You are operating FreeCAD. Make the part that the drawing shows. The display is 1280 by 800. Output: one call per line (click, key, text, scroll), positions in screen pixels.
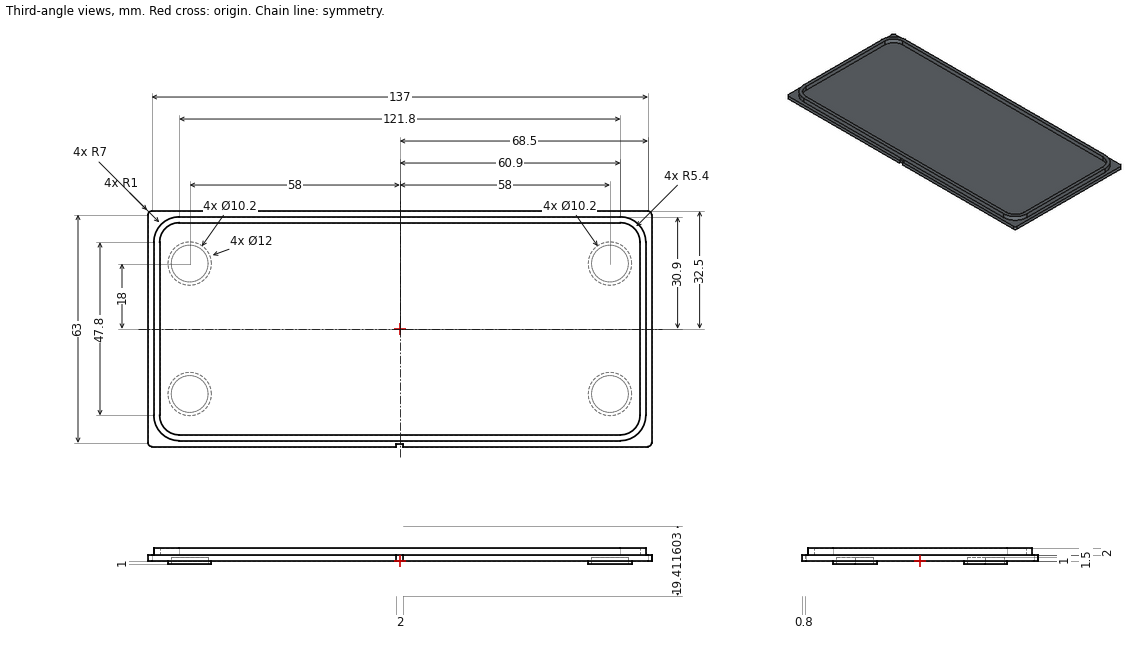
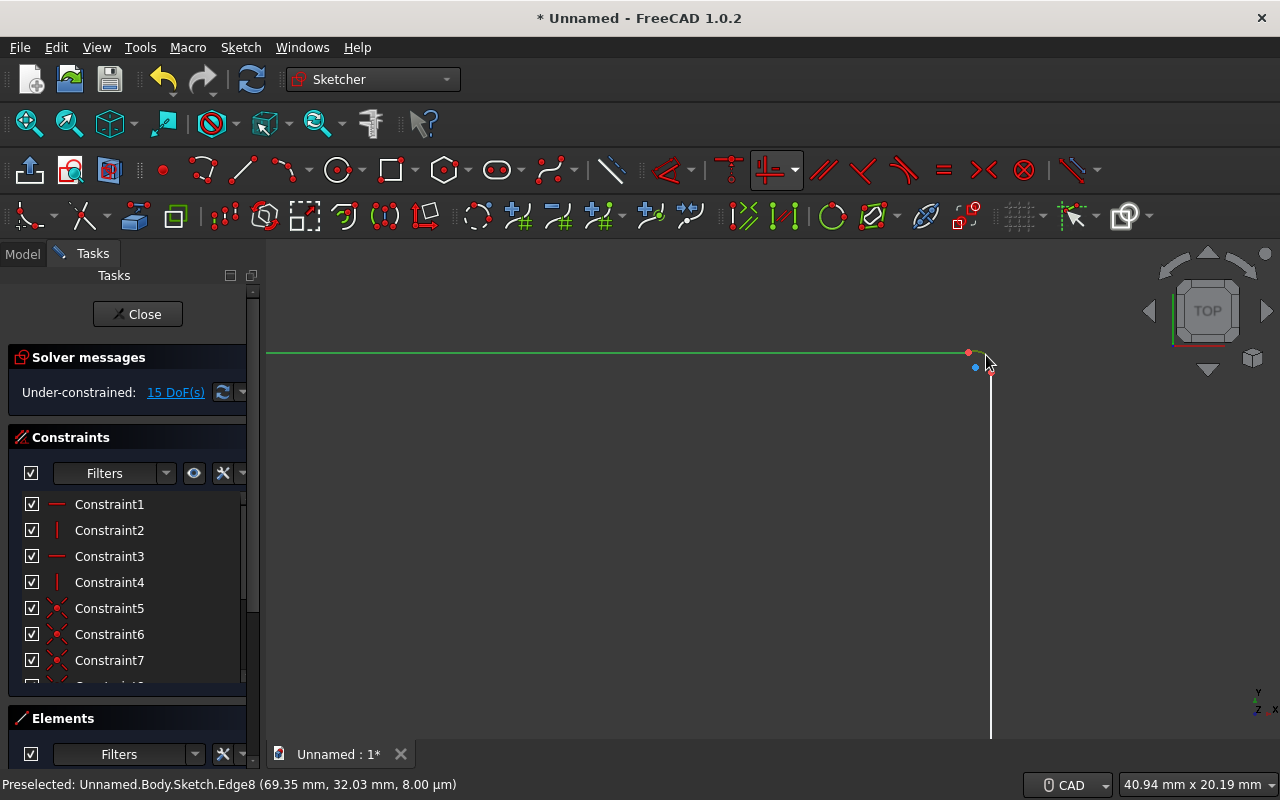
click(904, 170)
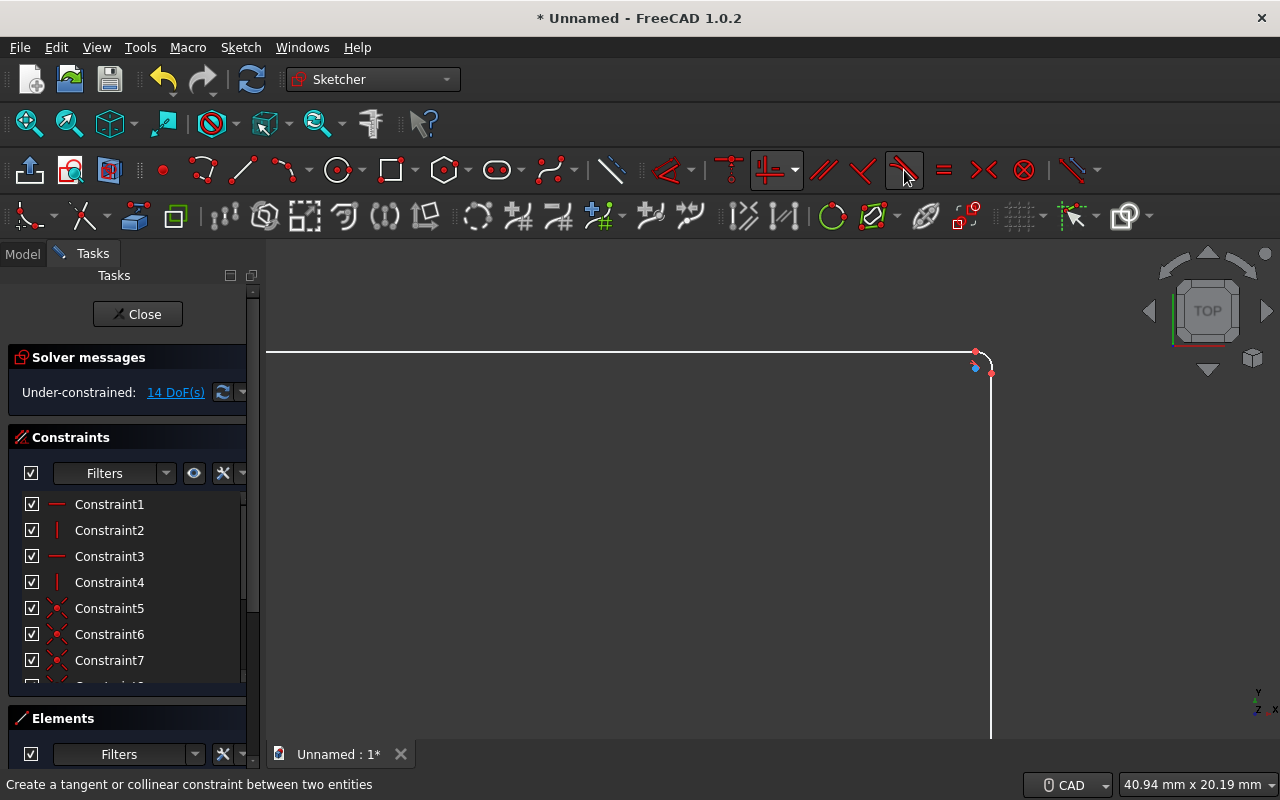
scroll(988, 358, down, 9)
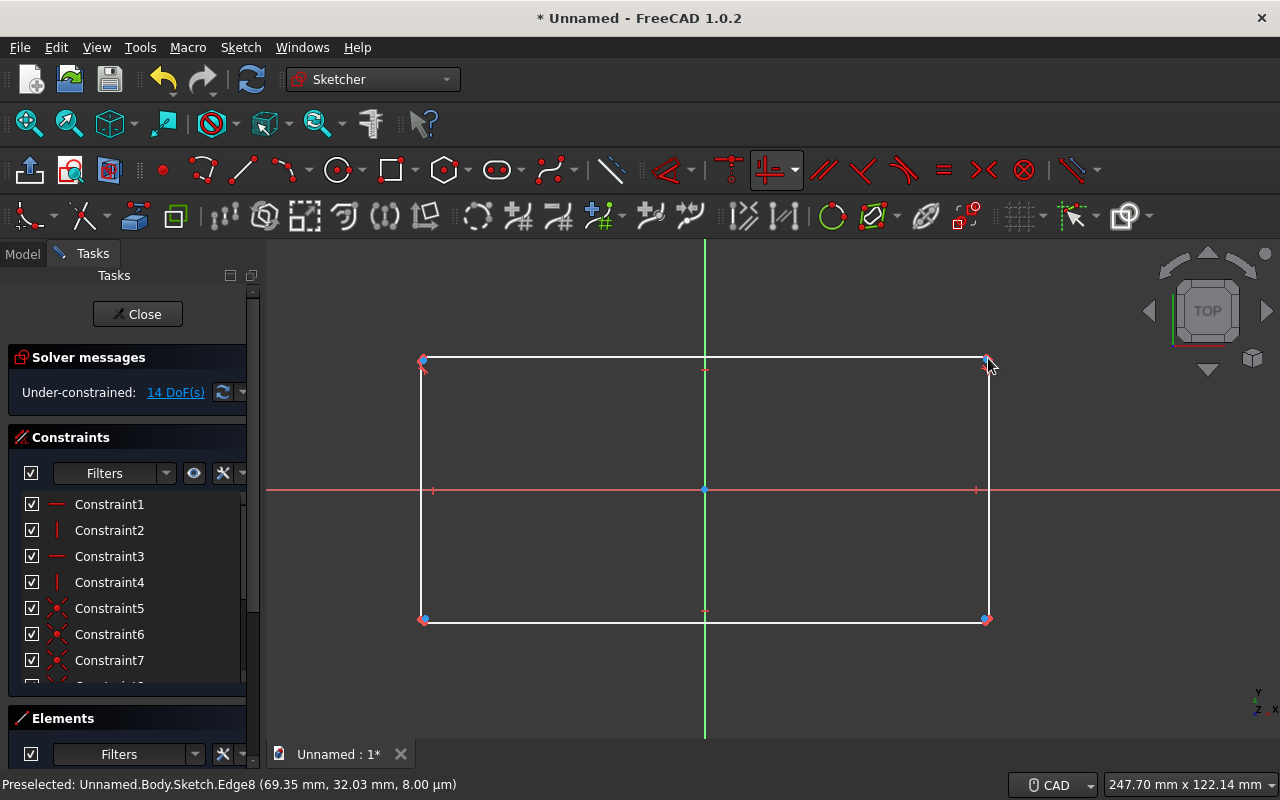
click(421, 439)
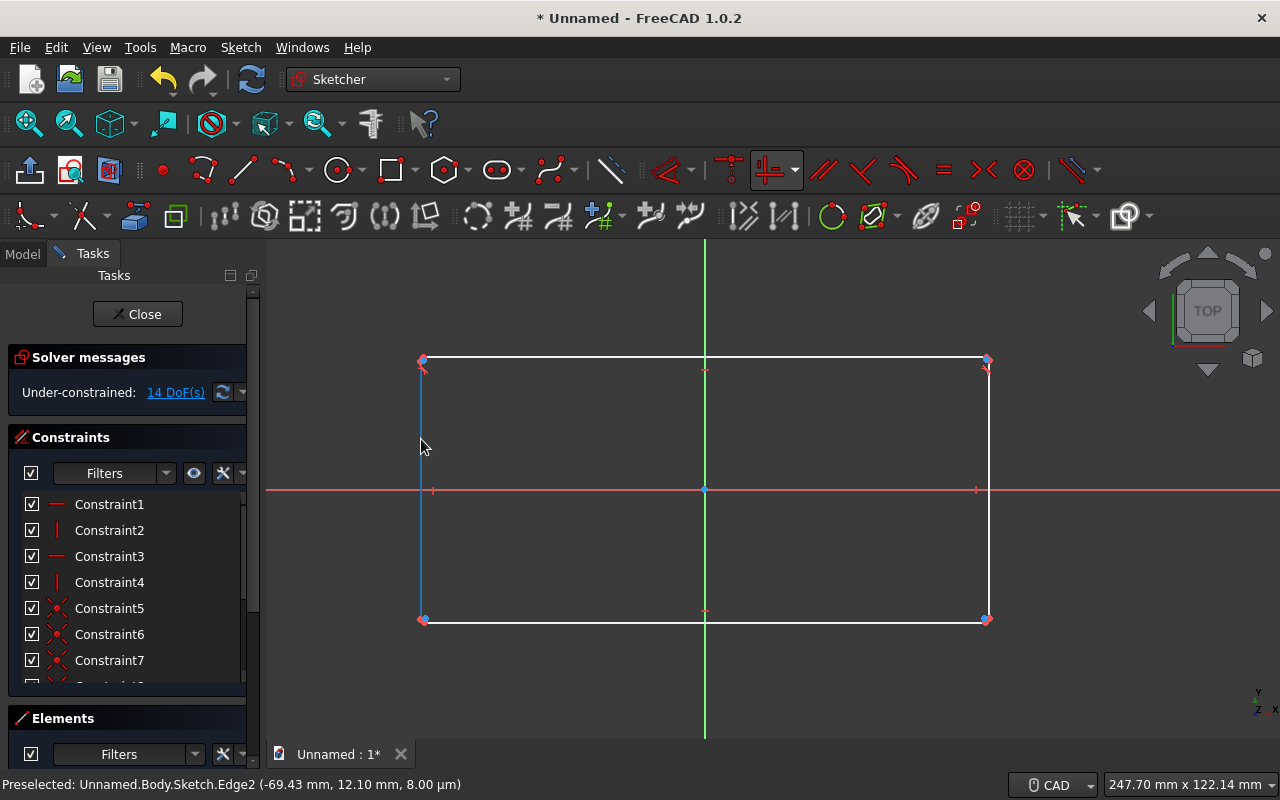
scroll(421, 358, up, 9)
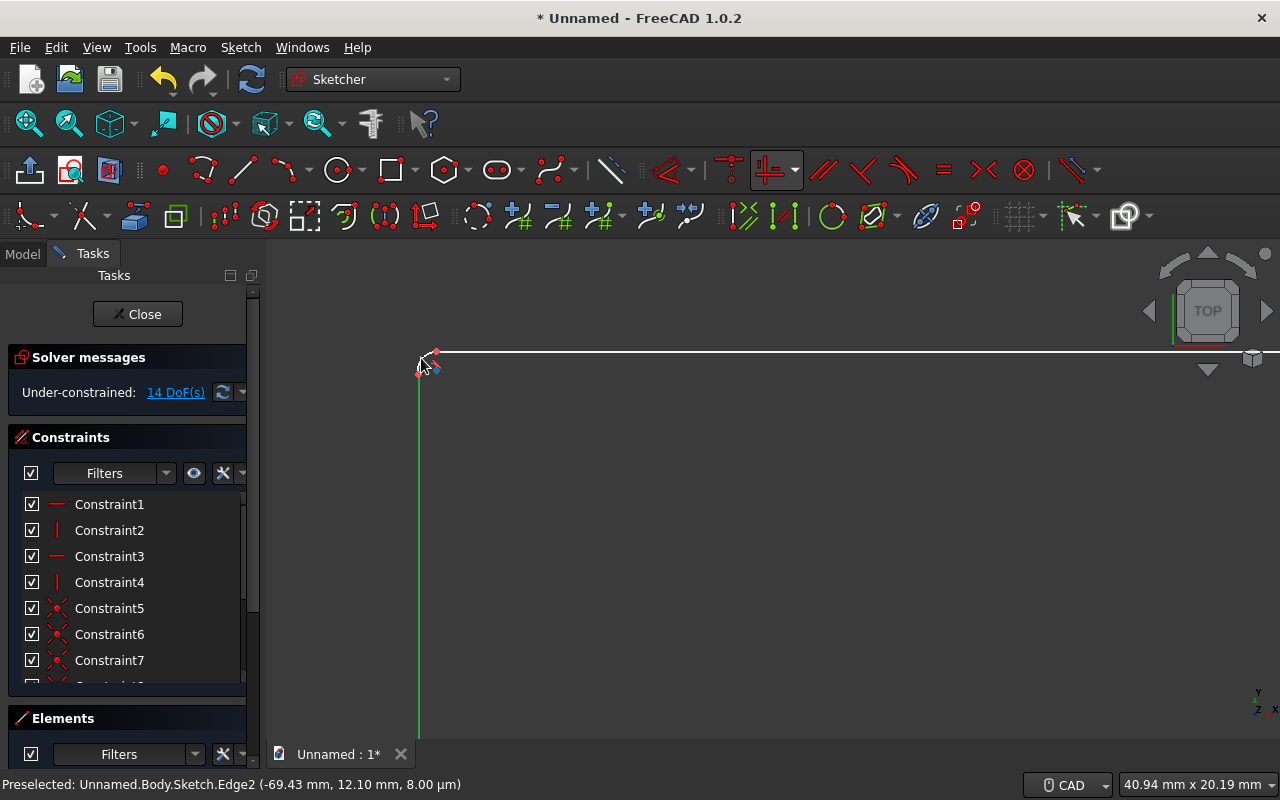
click(422, 359)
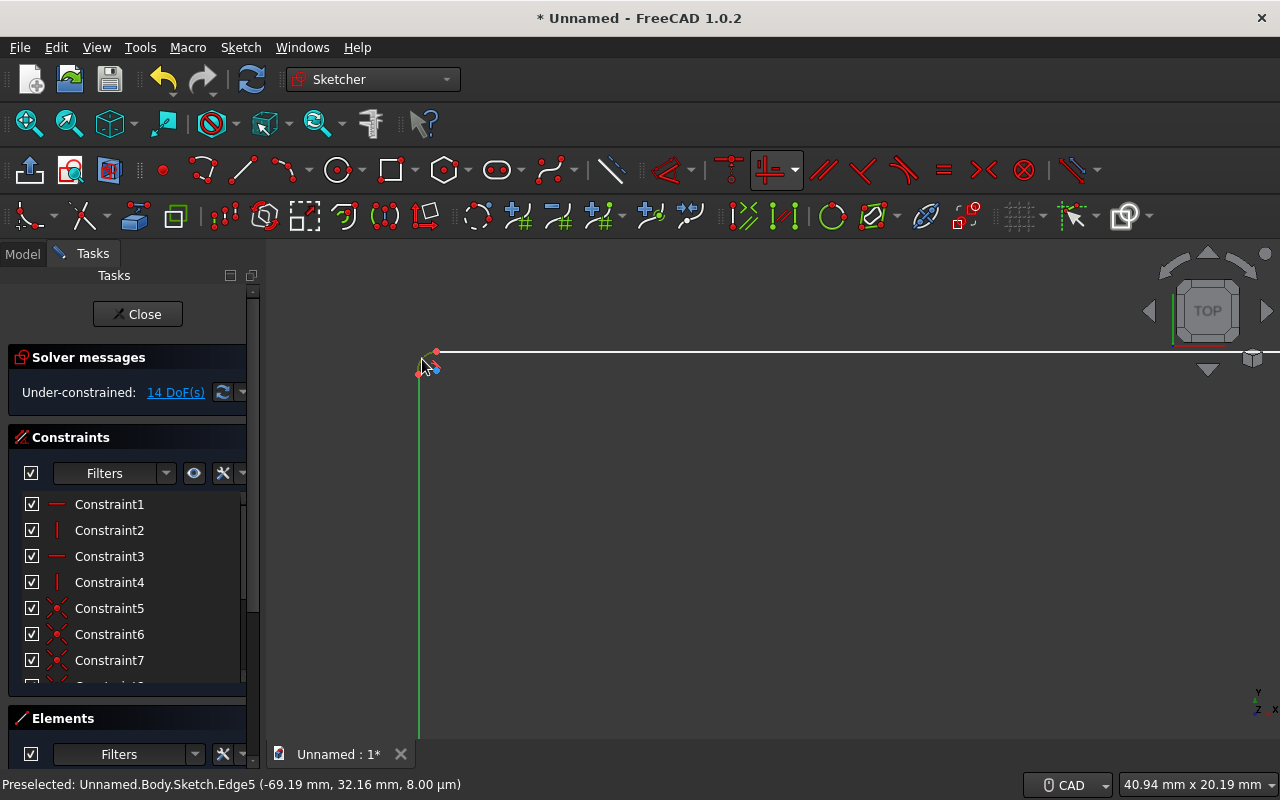
click(904, 170)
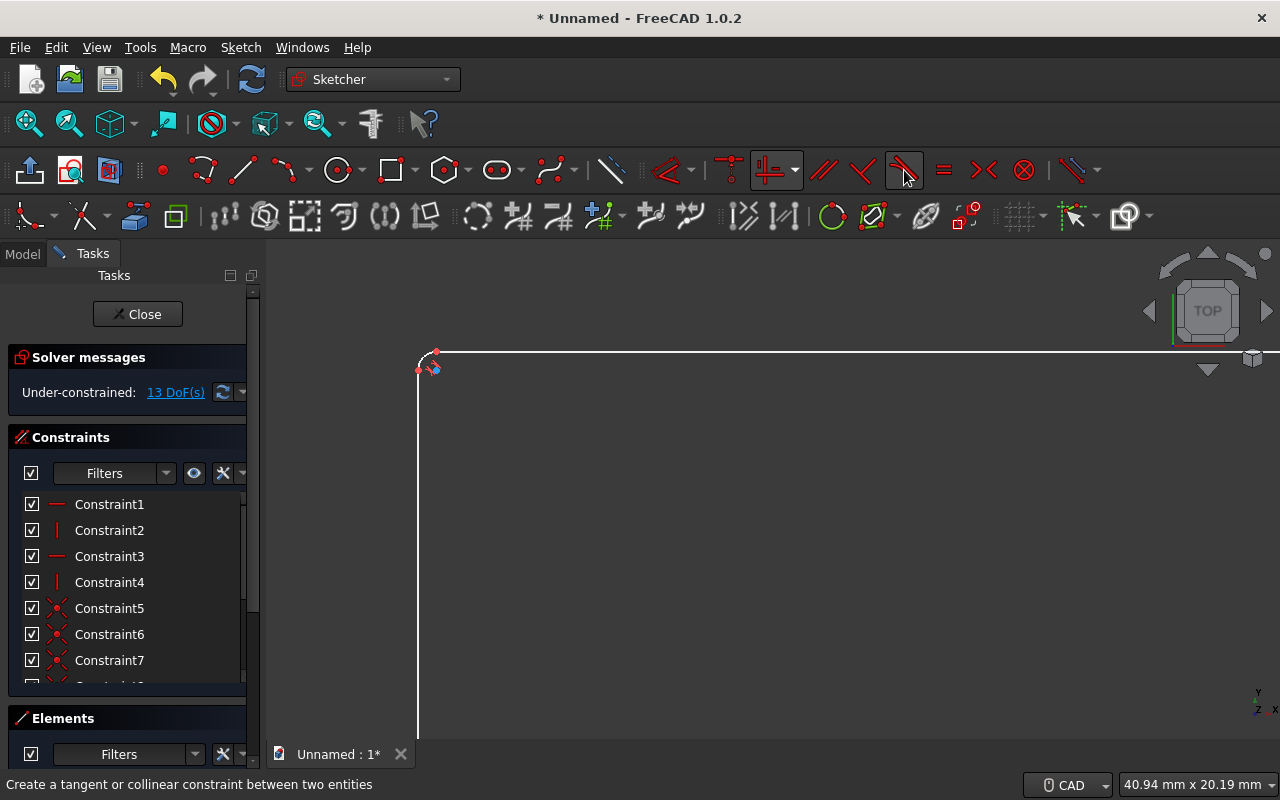
scroll(421, 358, down, 9)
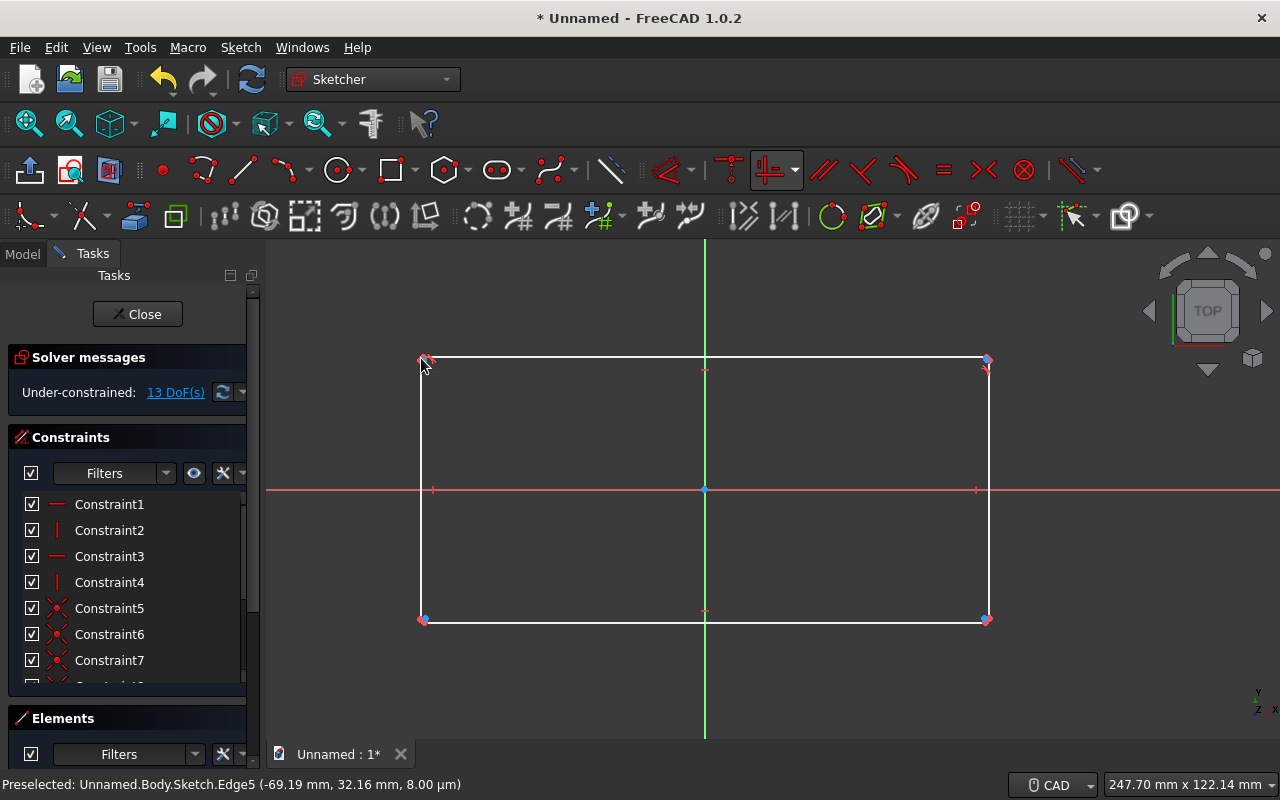
click(421, 412)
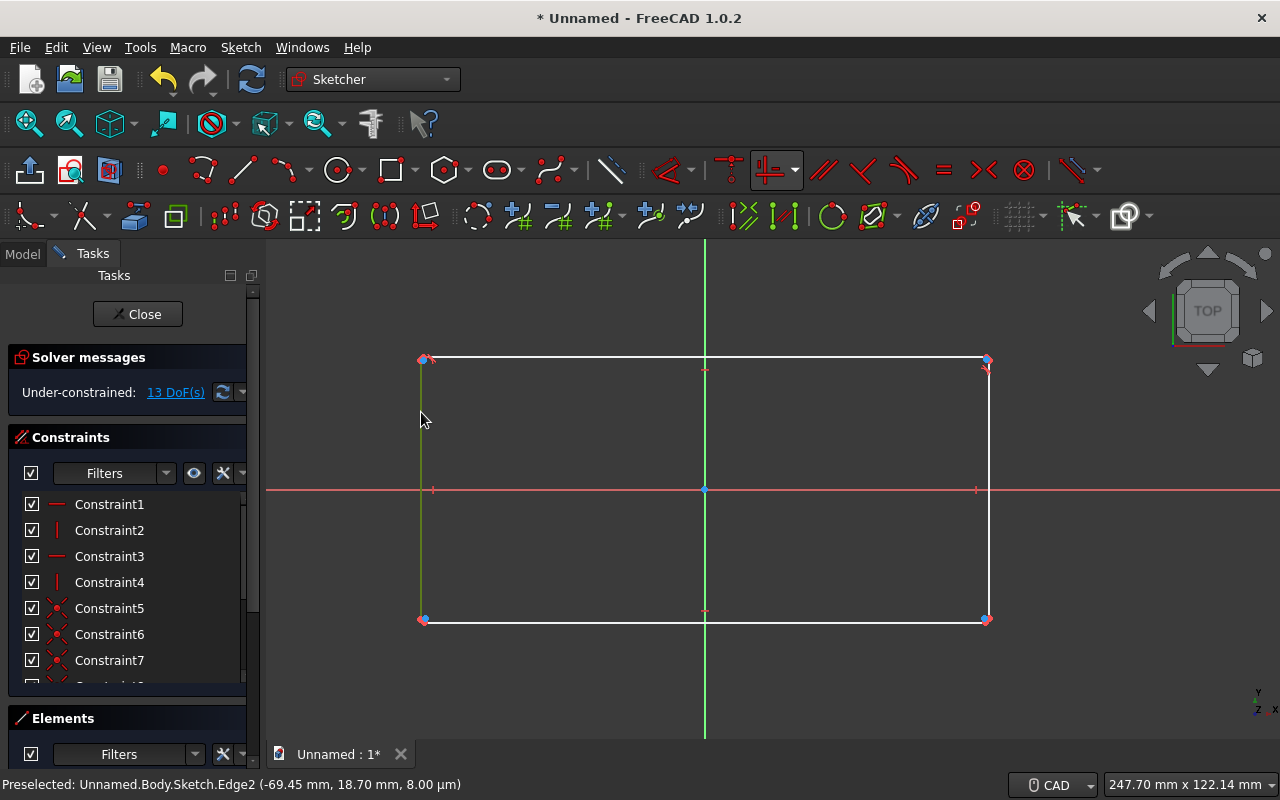
scroll(422, 622, up, 9)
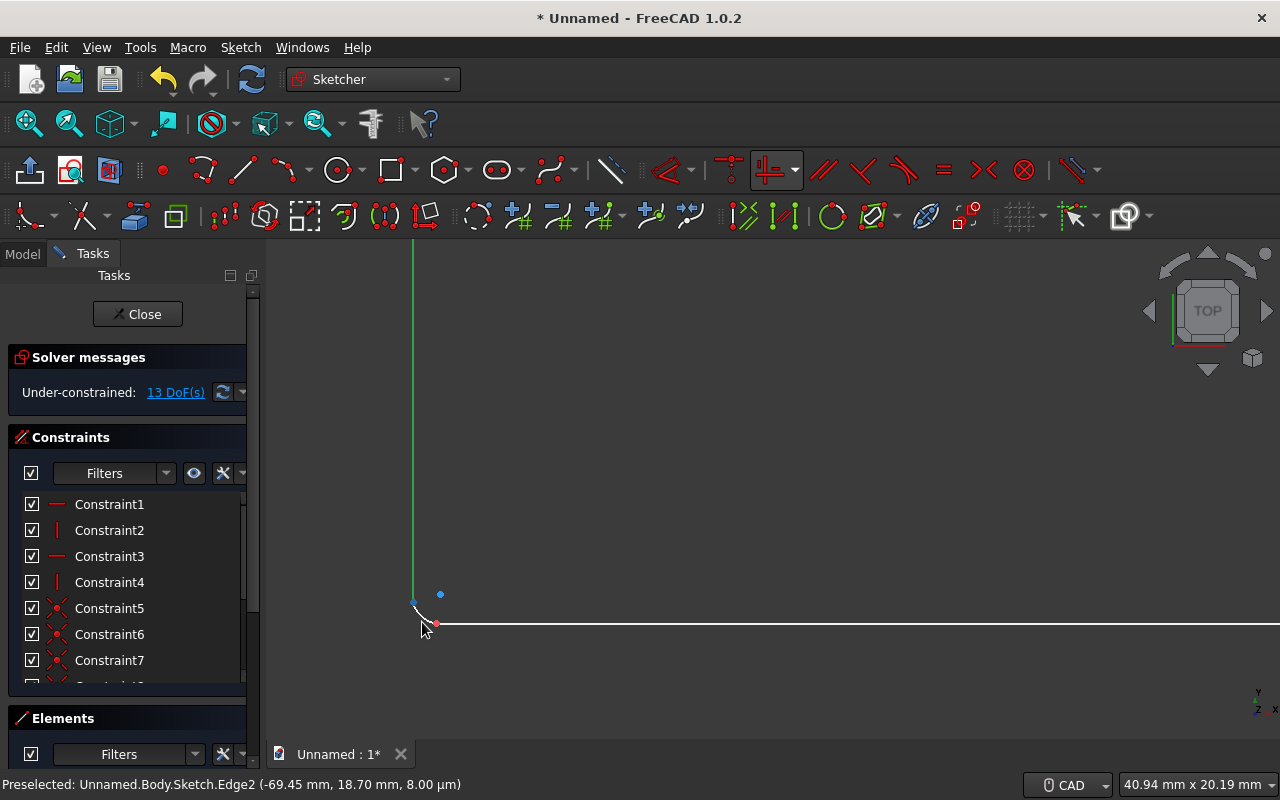
click(422, 617)